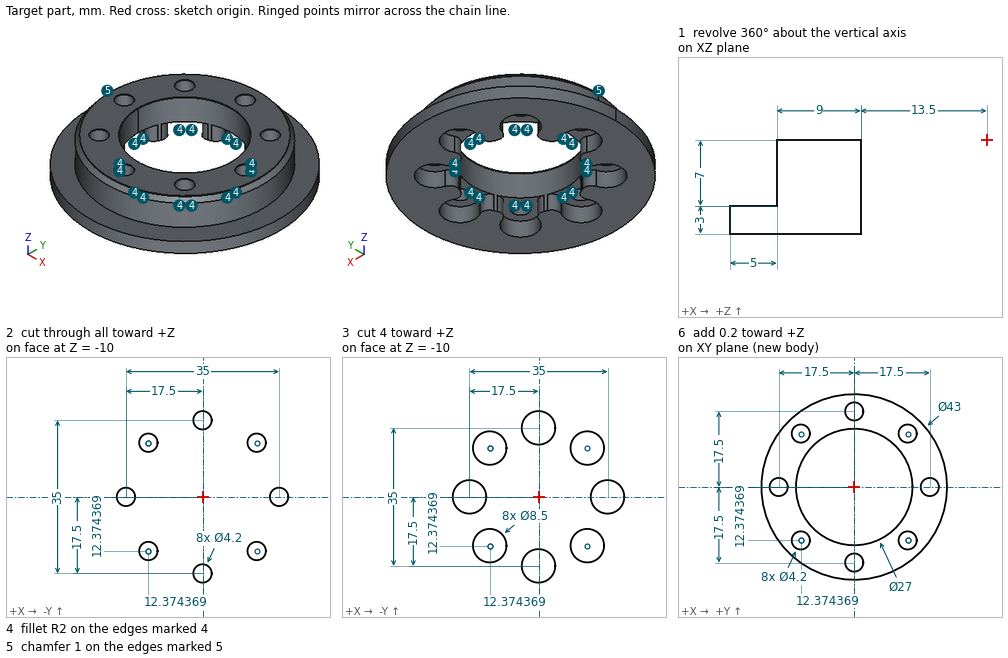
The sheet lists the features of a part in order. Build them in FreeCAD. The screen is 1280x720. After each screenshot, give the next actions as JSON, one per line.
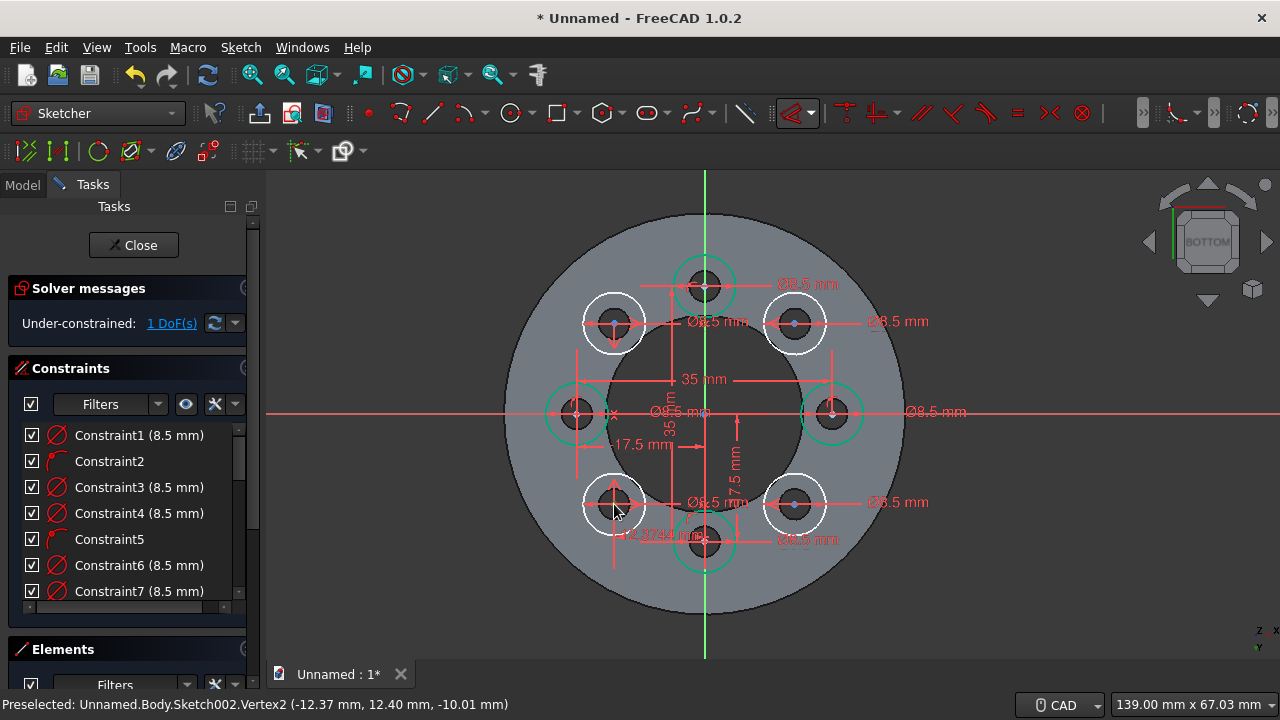
{"action": "key", "text": "i"}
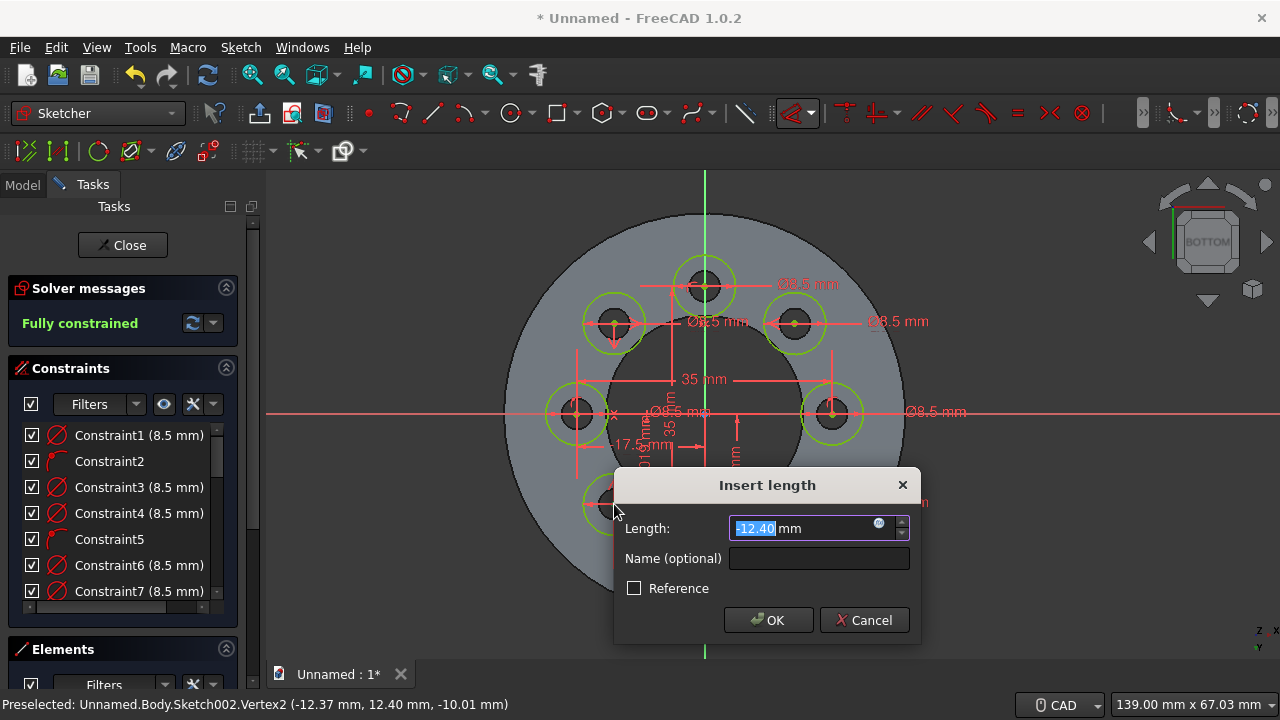
{"action": "type", "text": "-12.374369"}
{"action": "key", "text": "Return"}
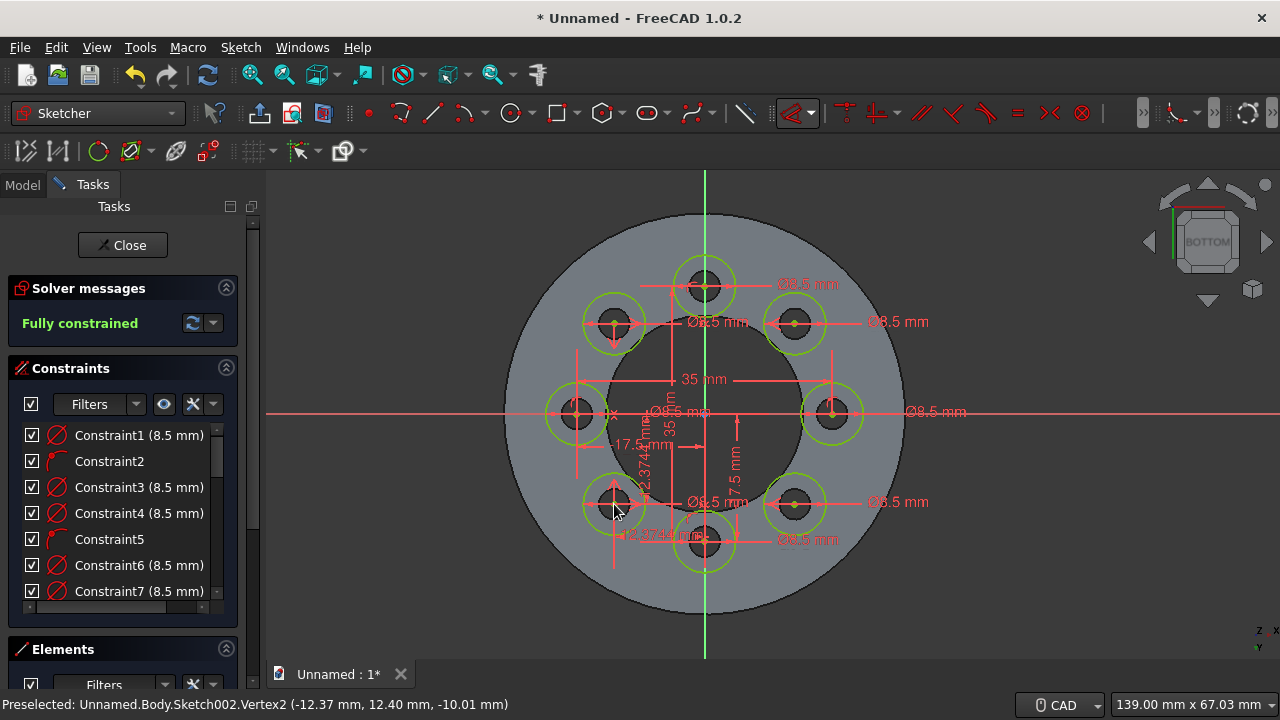
{"action": "left_click", "coordinate": [123, 245]}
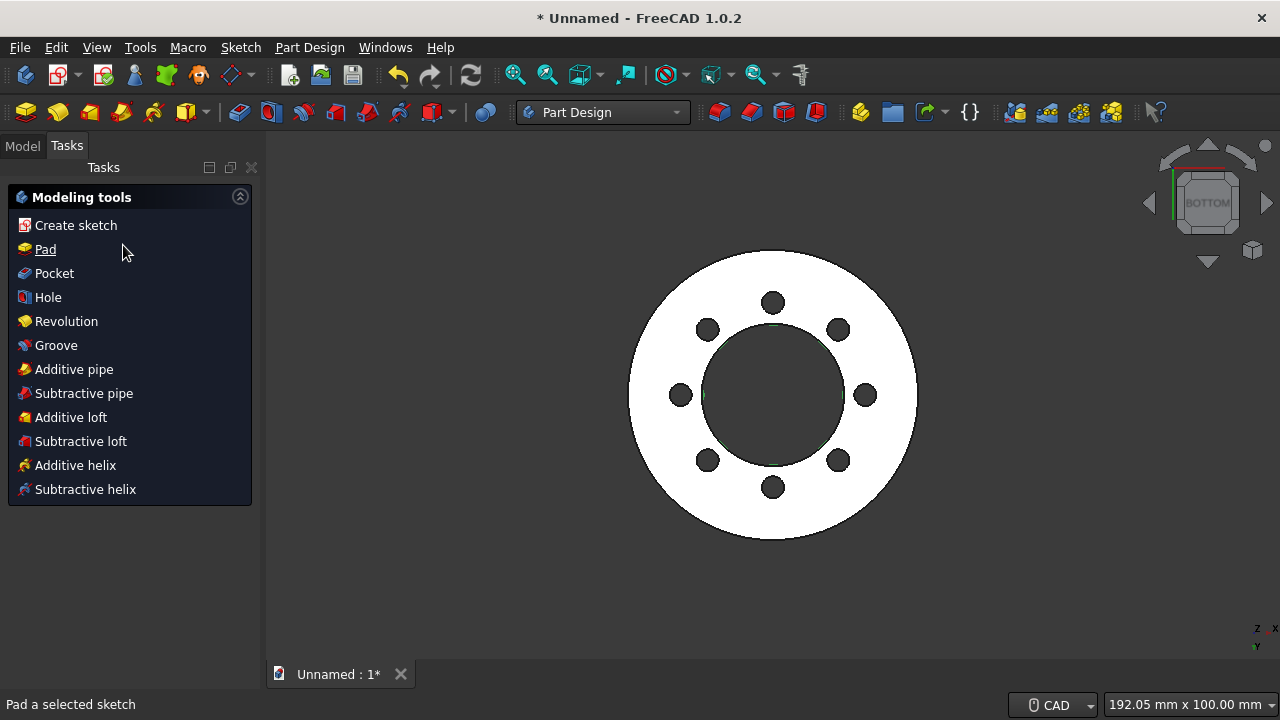
{"action": "left_click", "coordinate": [240, 112]}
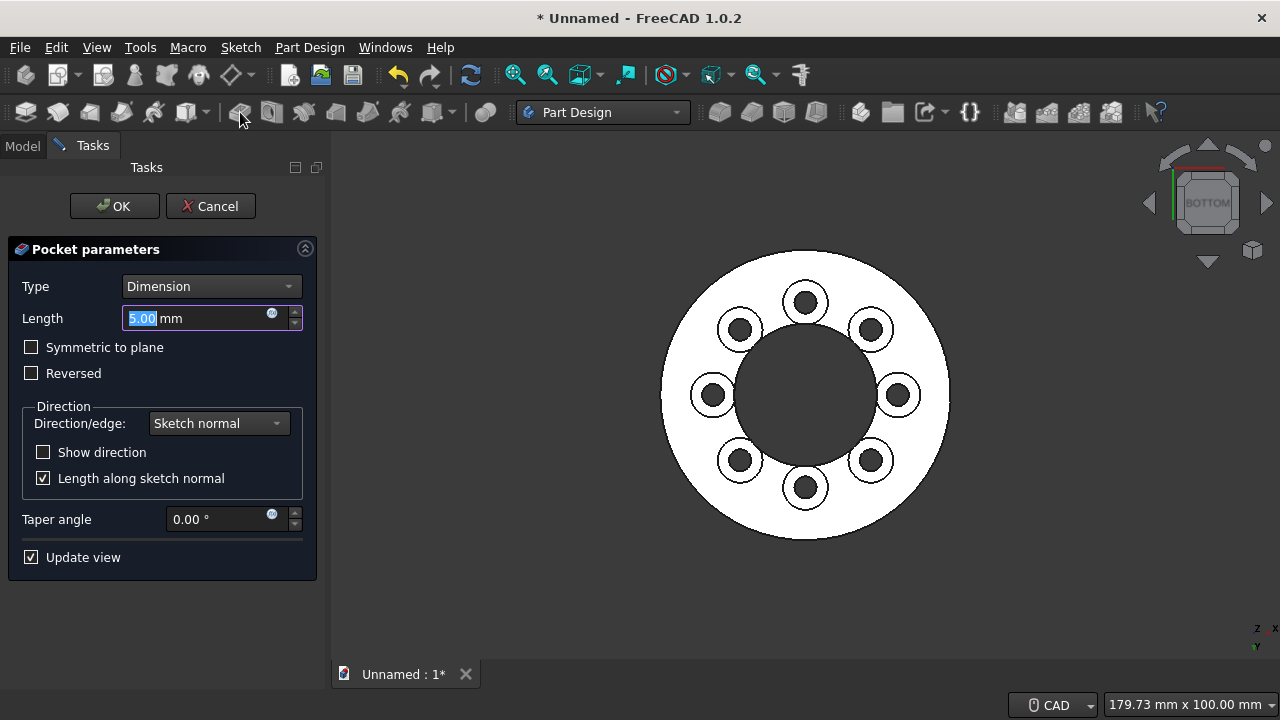
{"action": "type", "text": "4"}
{"action": "key", "text": "Tab"}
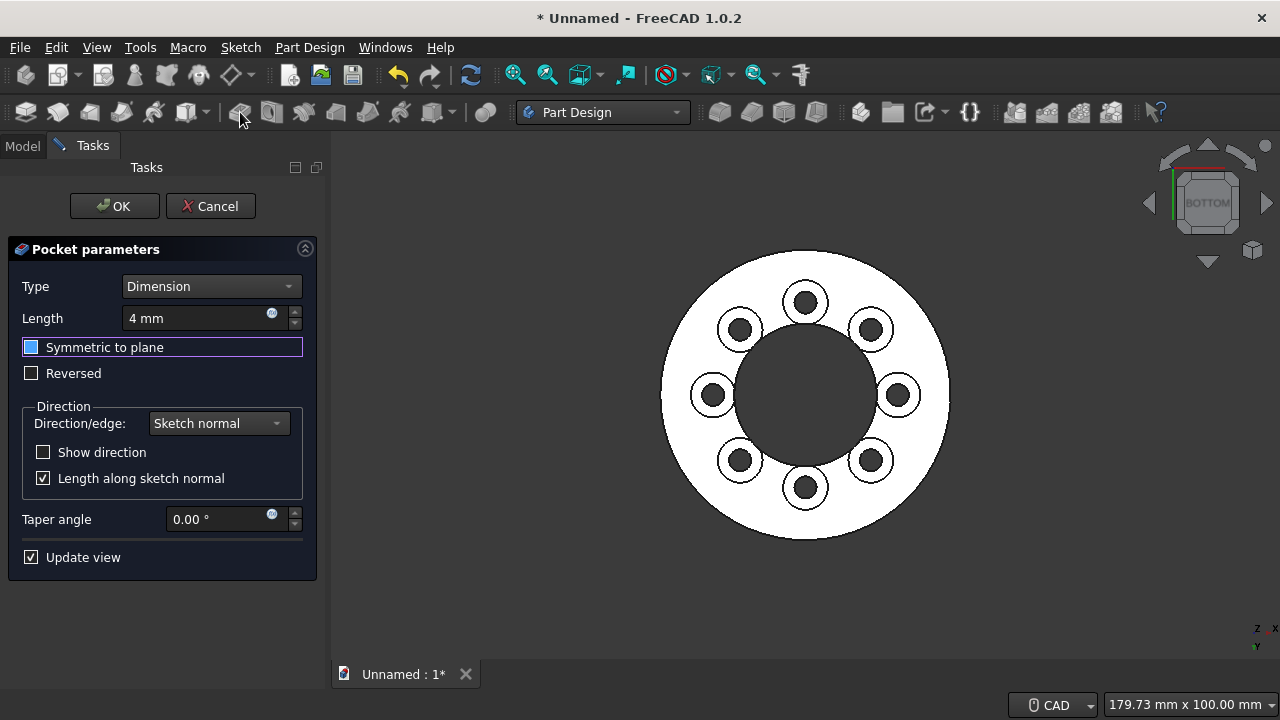
{"action": "left_click", "coordinate": [115, 206]}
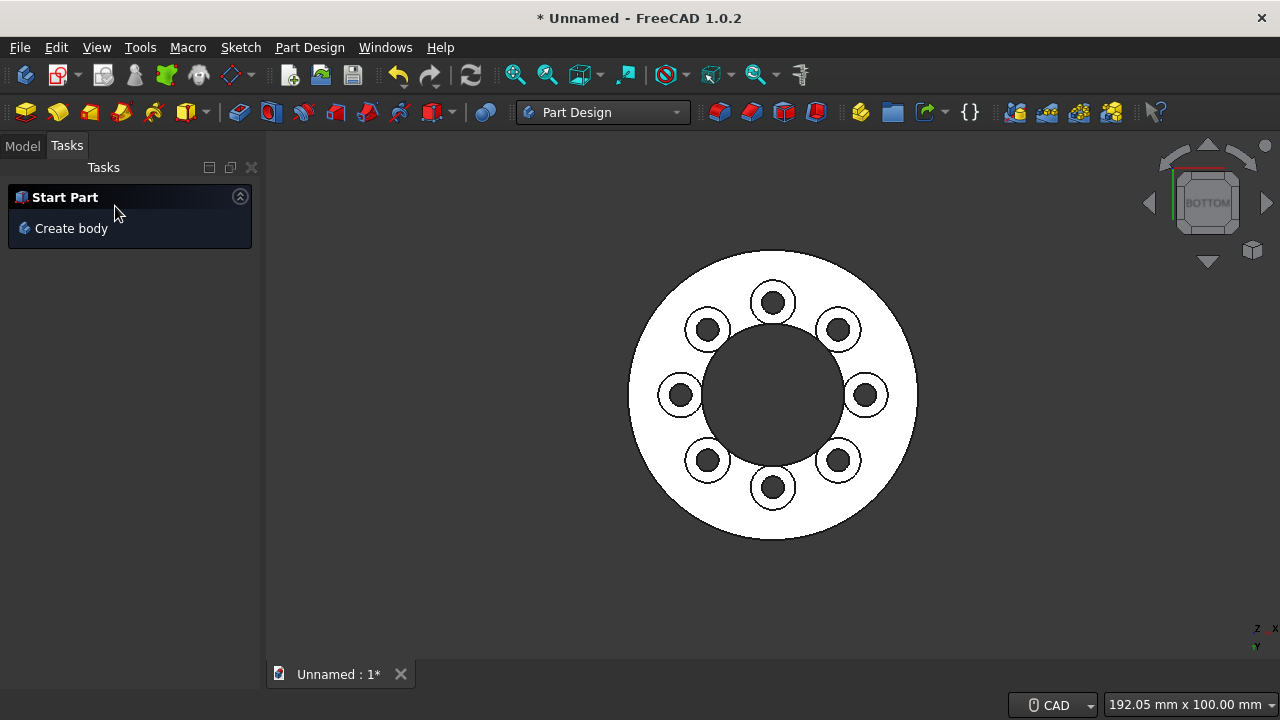
{"action": "scroll", "coordinate": [780, 465], "scroll_direction": "up", "scroll_amount": 4}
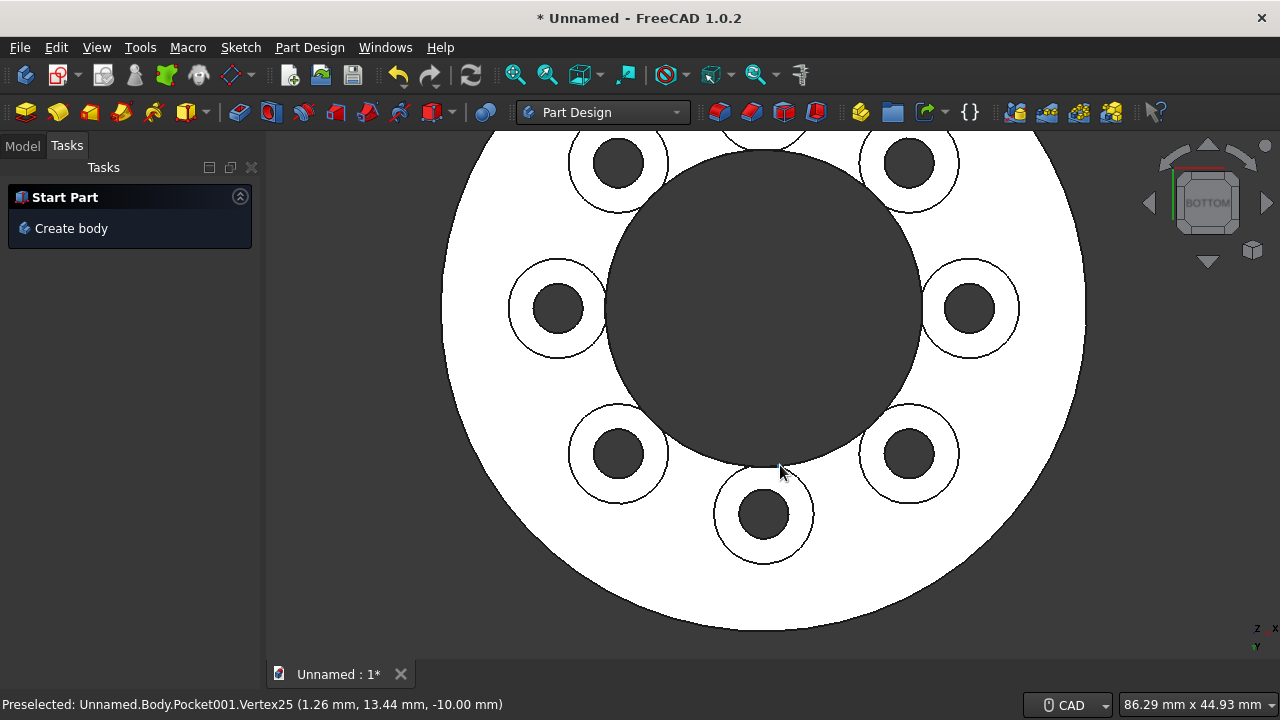
{"action": "key", "text": "v f"}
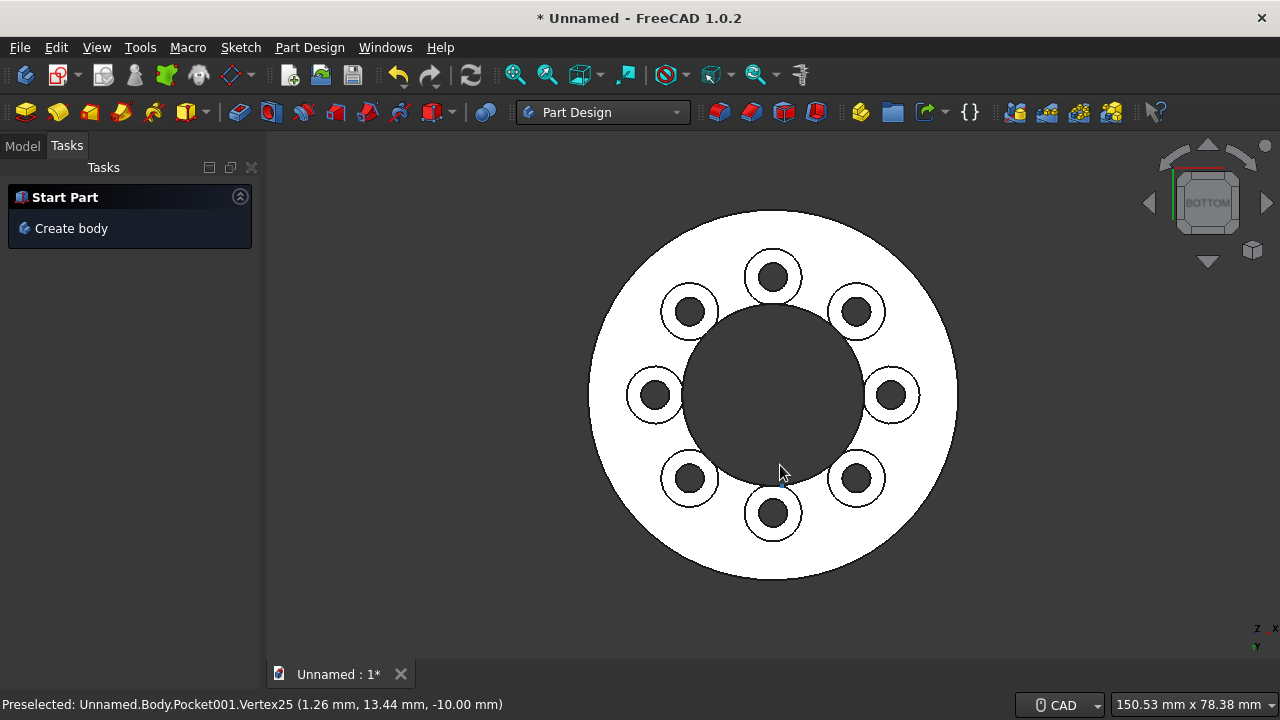
{"action": "key", "text": "0"}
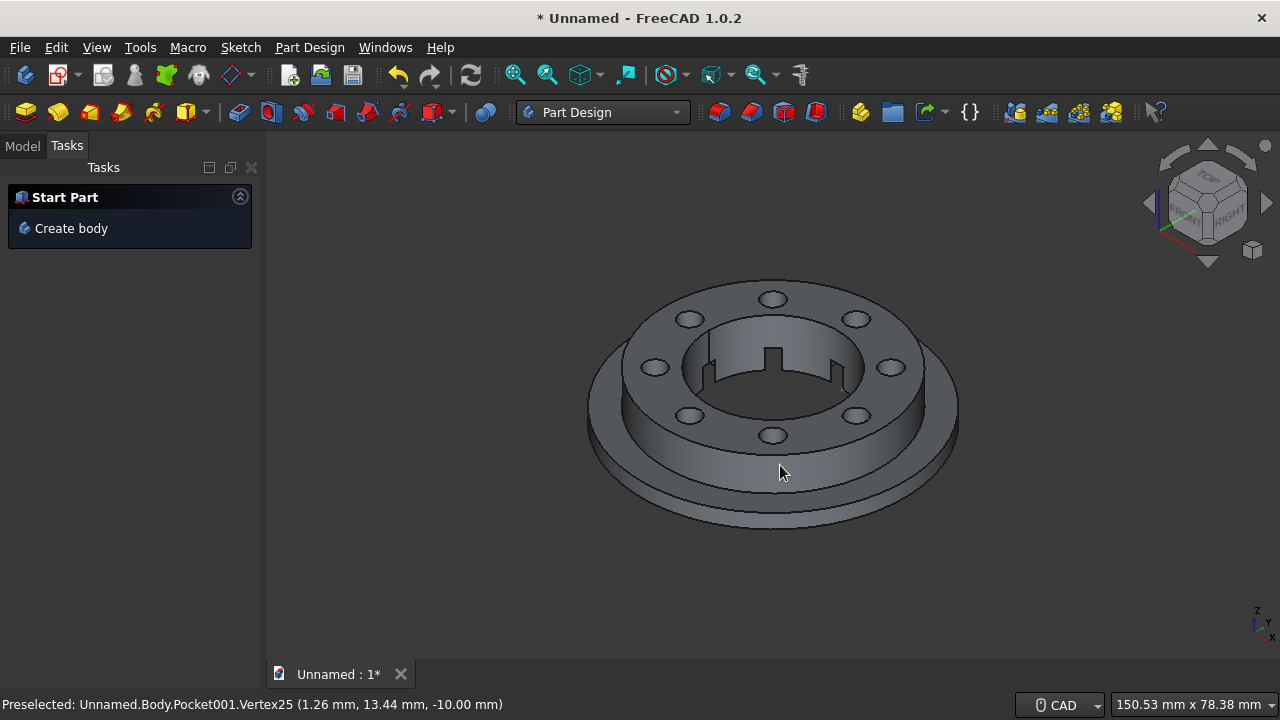
{"action": "left_click", "coordinate": [831, 370]}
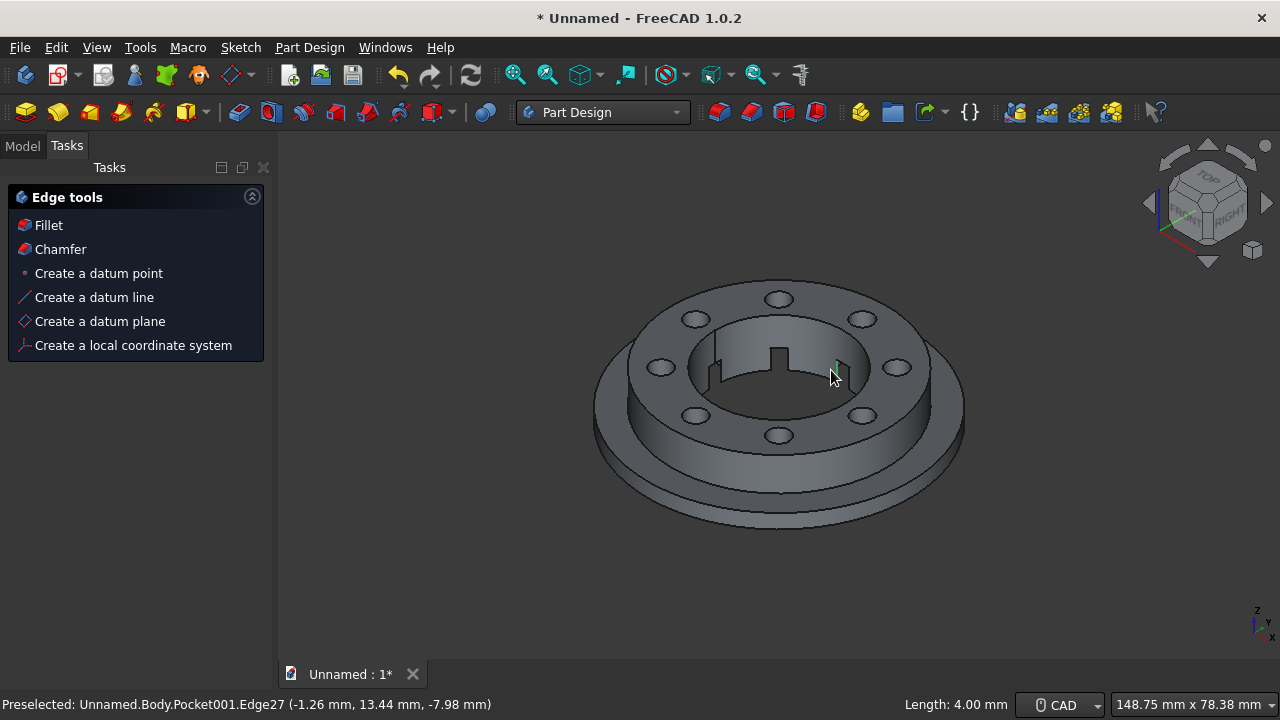
{"action": "left_click", "coordinate": [721, 370], "text": "ctrl"}